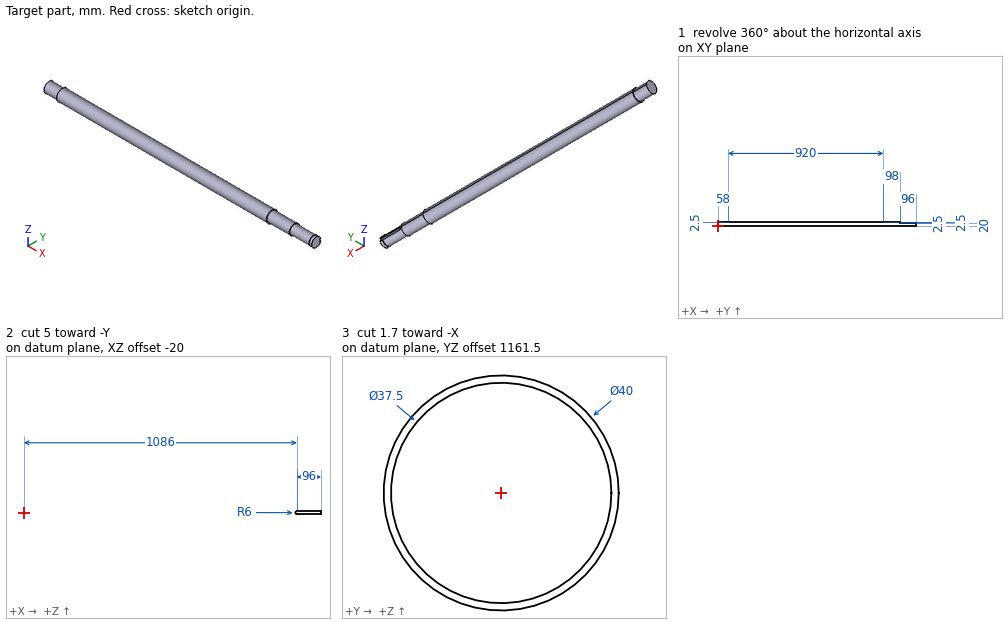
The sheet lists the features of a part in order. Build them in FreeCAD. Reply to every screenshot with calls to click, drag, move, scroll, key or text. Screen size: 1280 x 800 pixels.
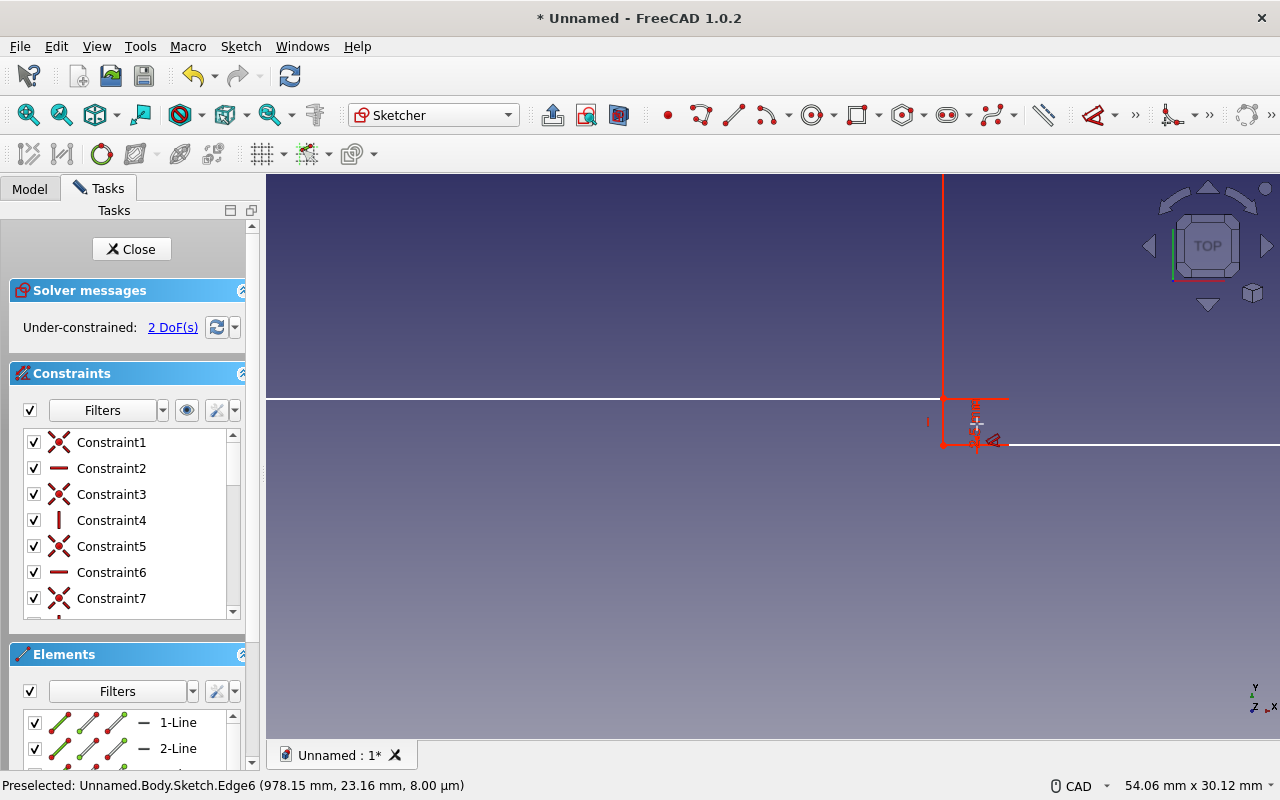
scroll(950, 450, down, 17)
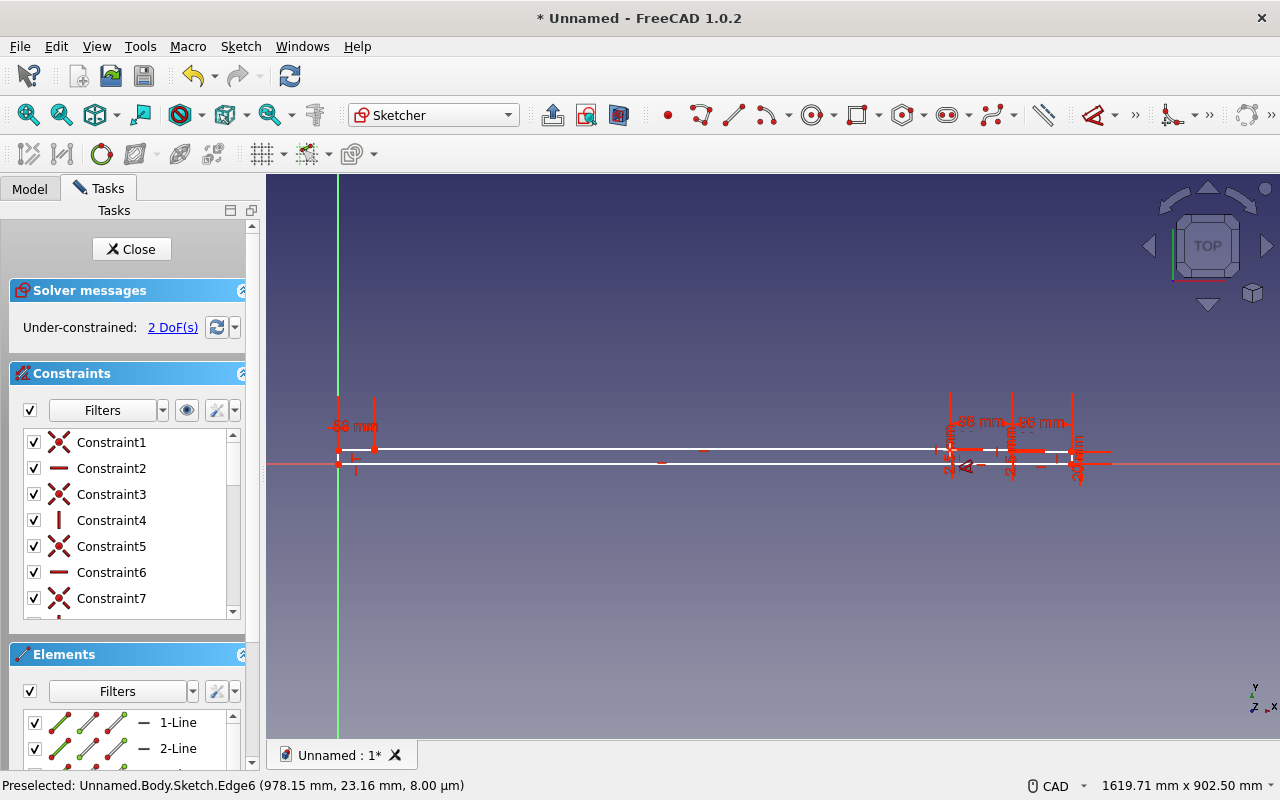
click(778, 449)
click(662, 415)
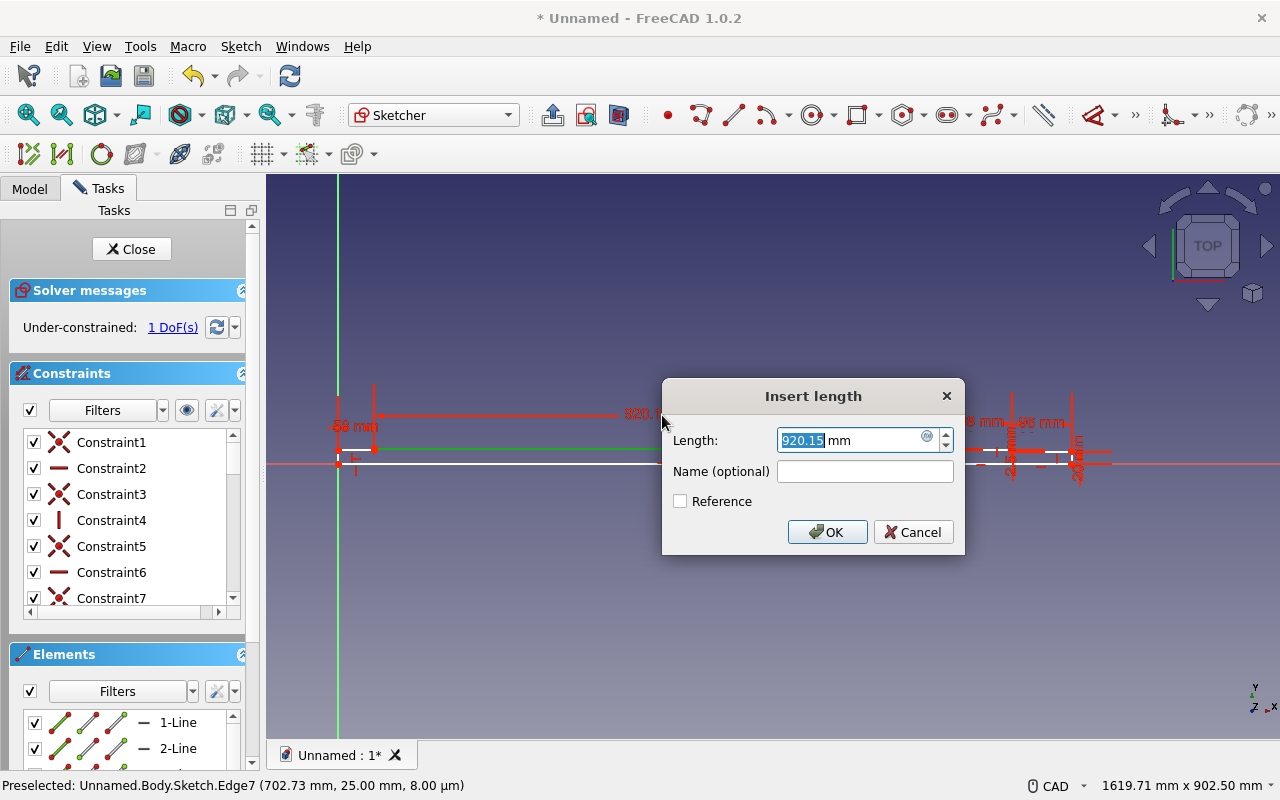
text(920)
key(Return)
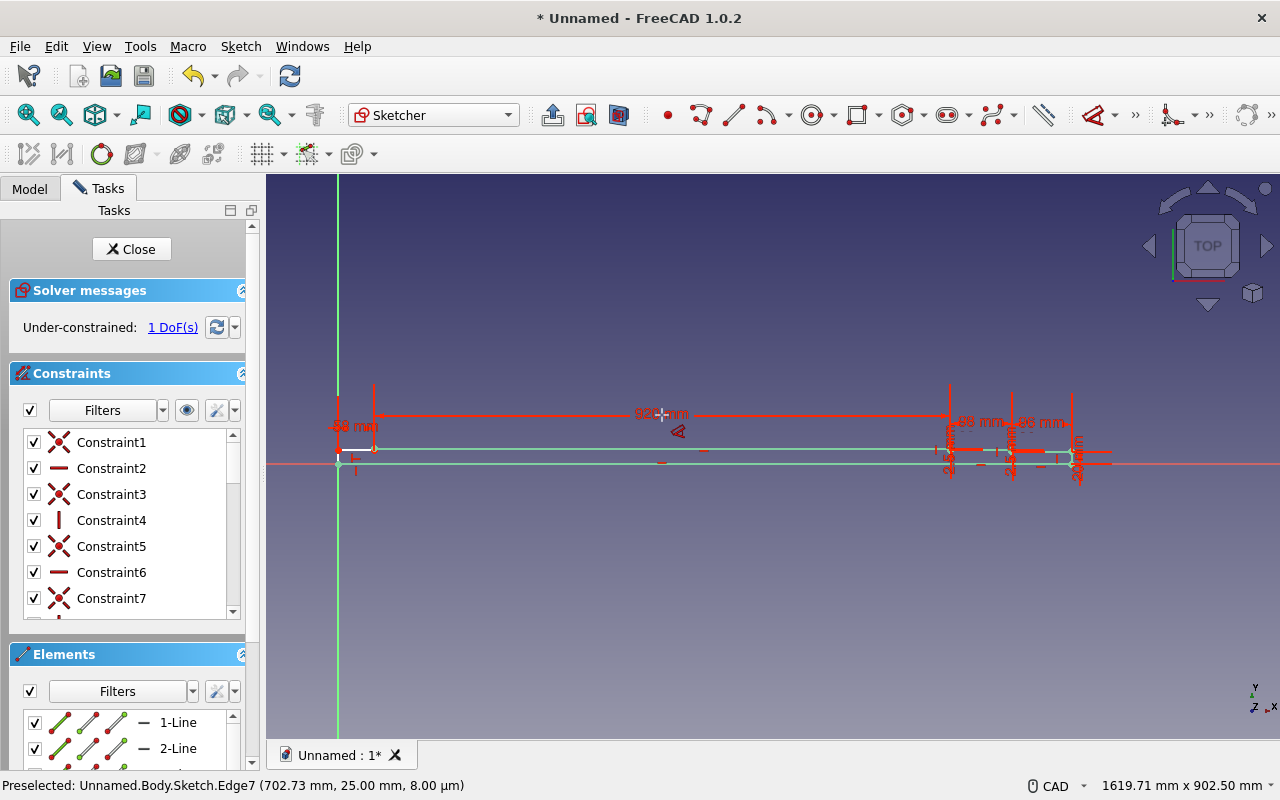
scroll(374, 450, up, 17)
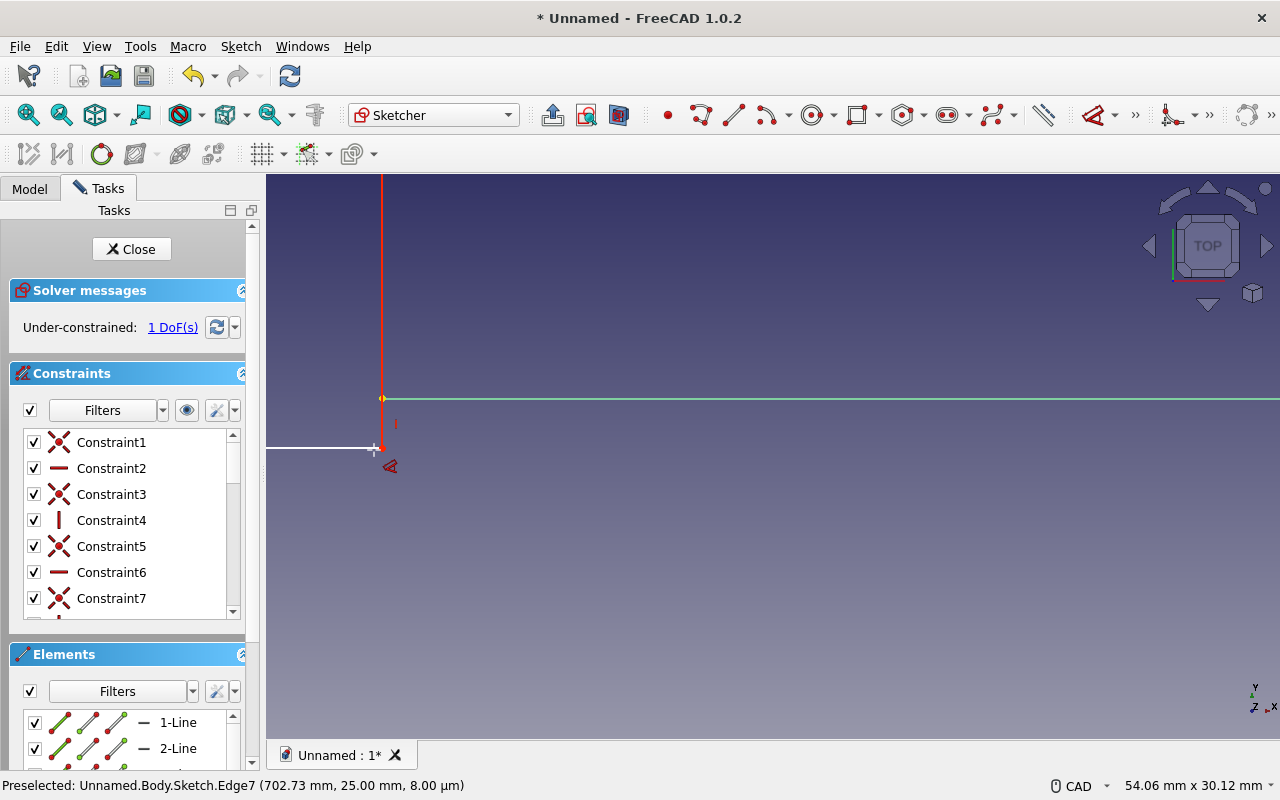
click(382, 423)
click(348, 423)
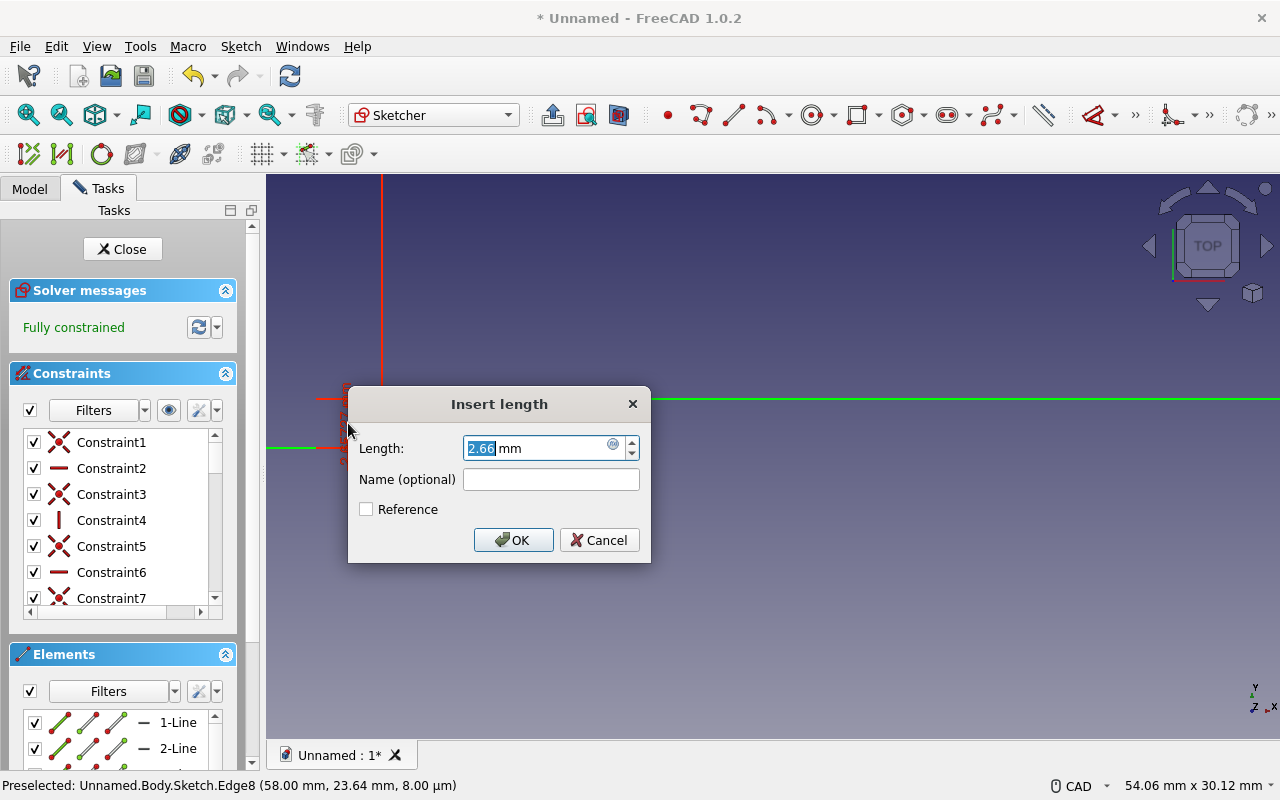
text(2.5)
key(Return)
key(Escape)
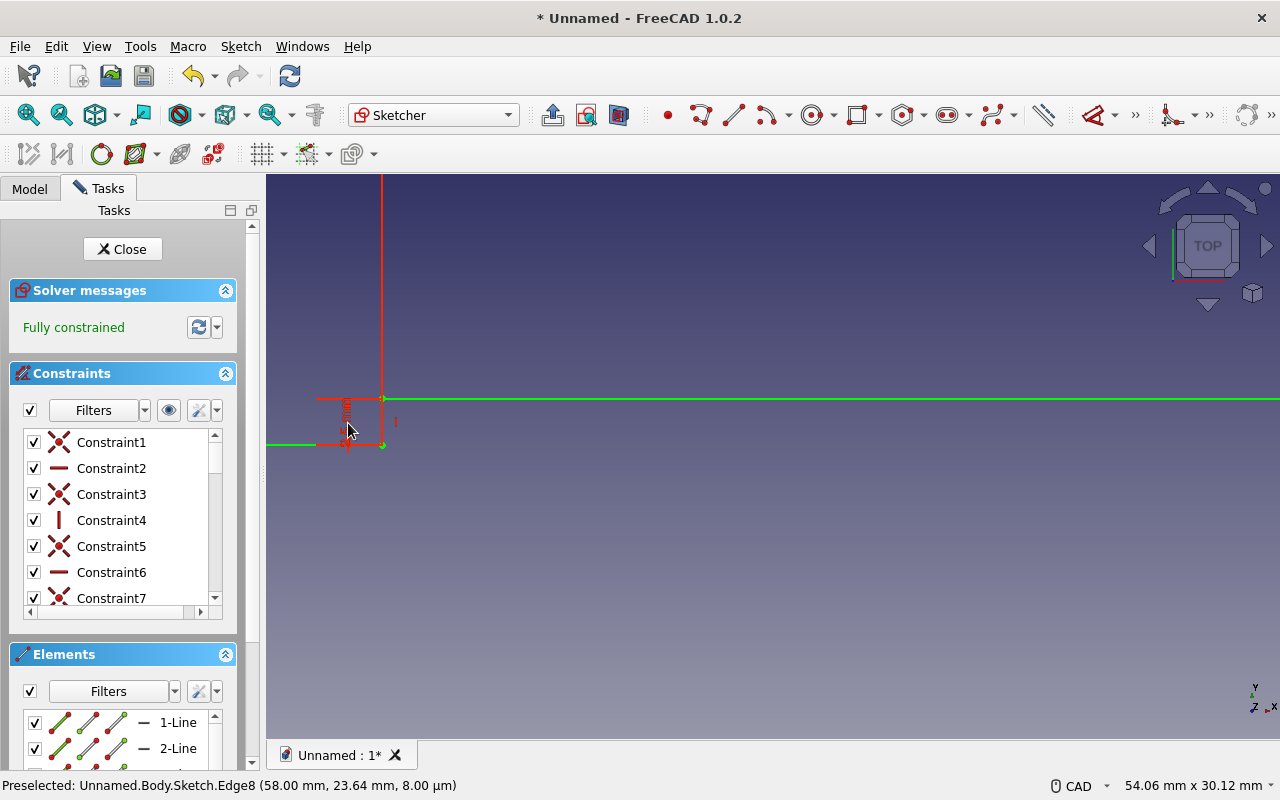
click(123, 249)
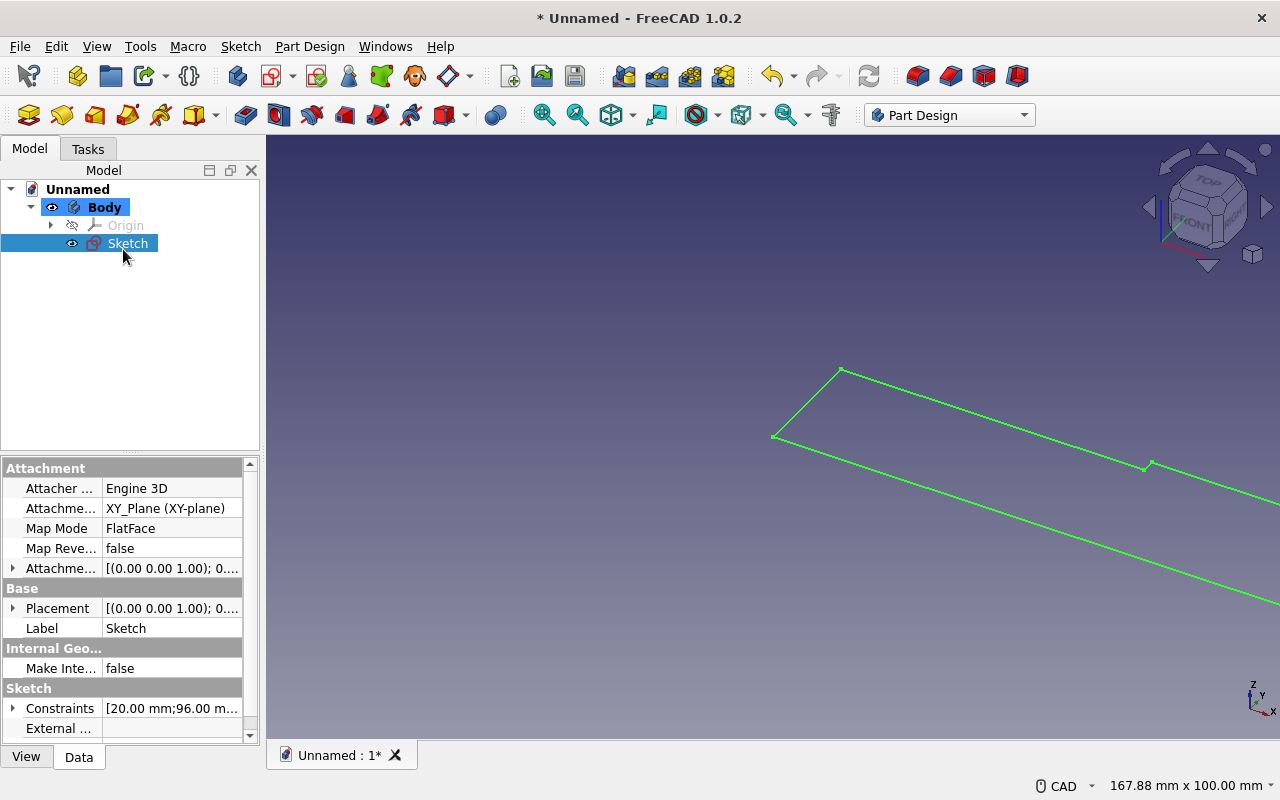
click(62, 116)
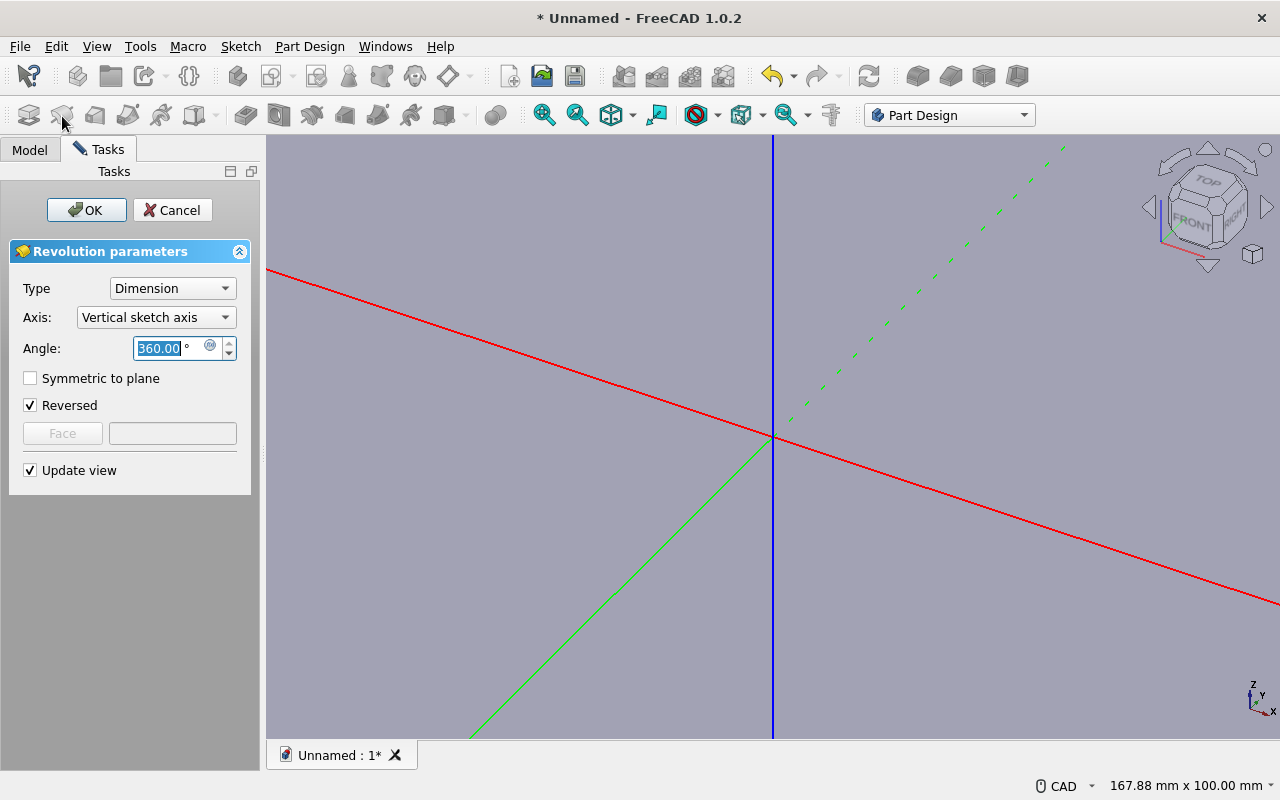
click(157, 318)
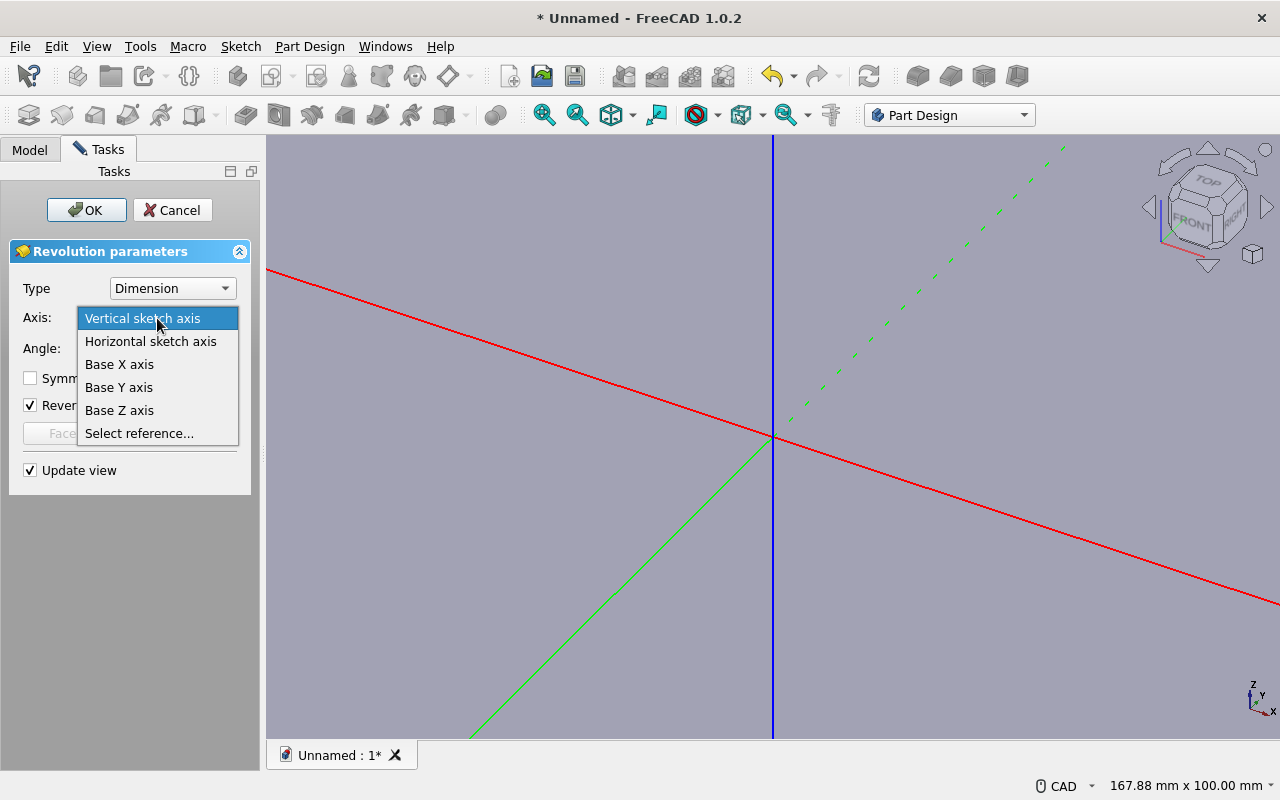
click(156, 342)